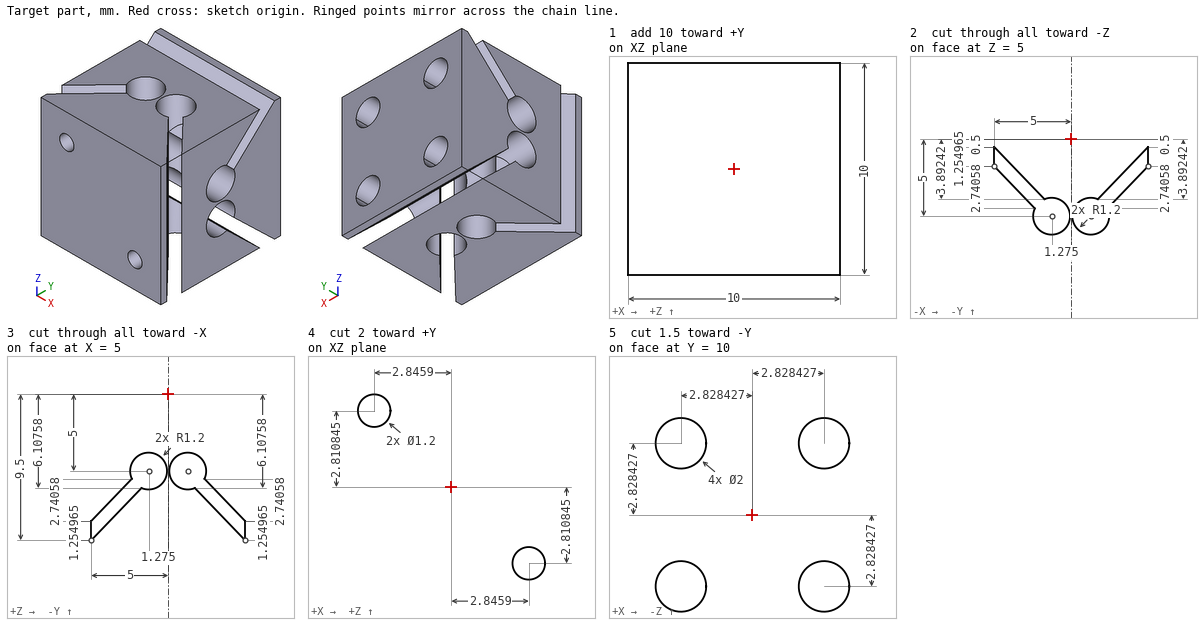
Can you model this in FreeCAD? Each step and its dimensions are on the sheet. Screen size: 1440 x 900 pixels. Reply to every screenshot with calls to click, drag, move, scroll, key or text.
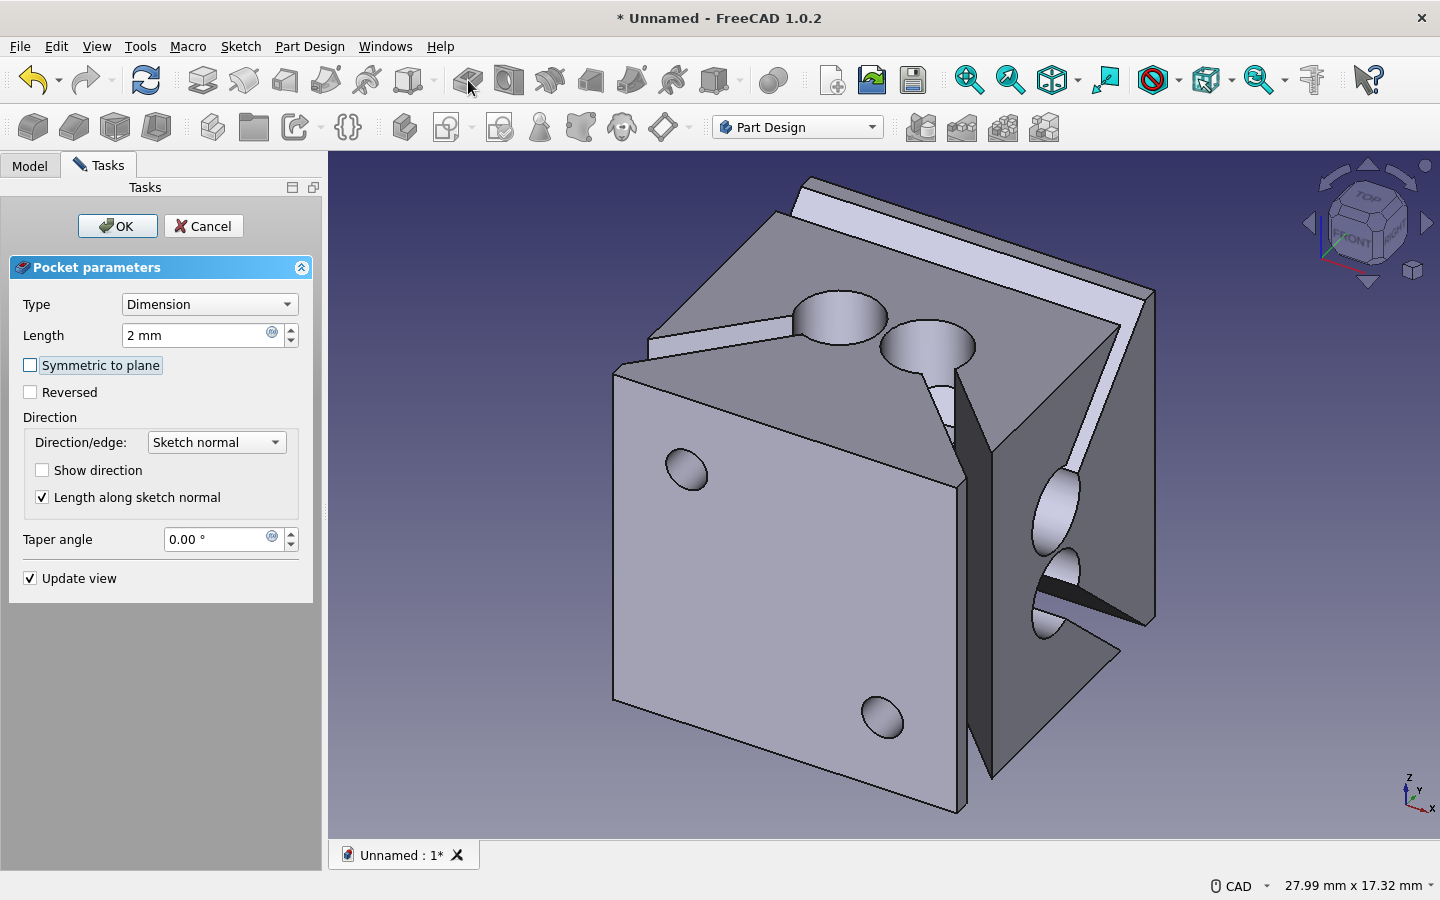
click(118, 226)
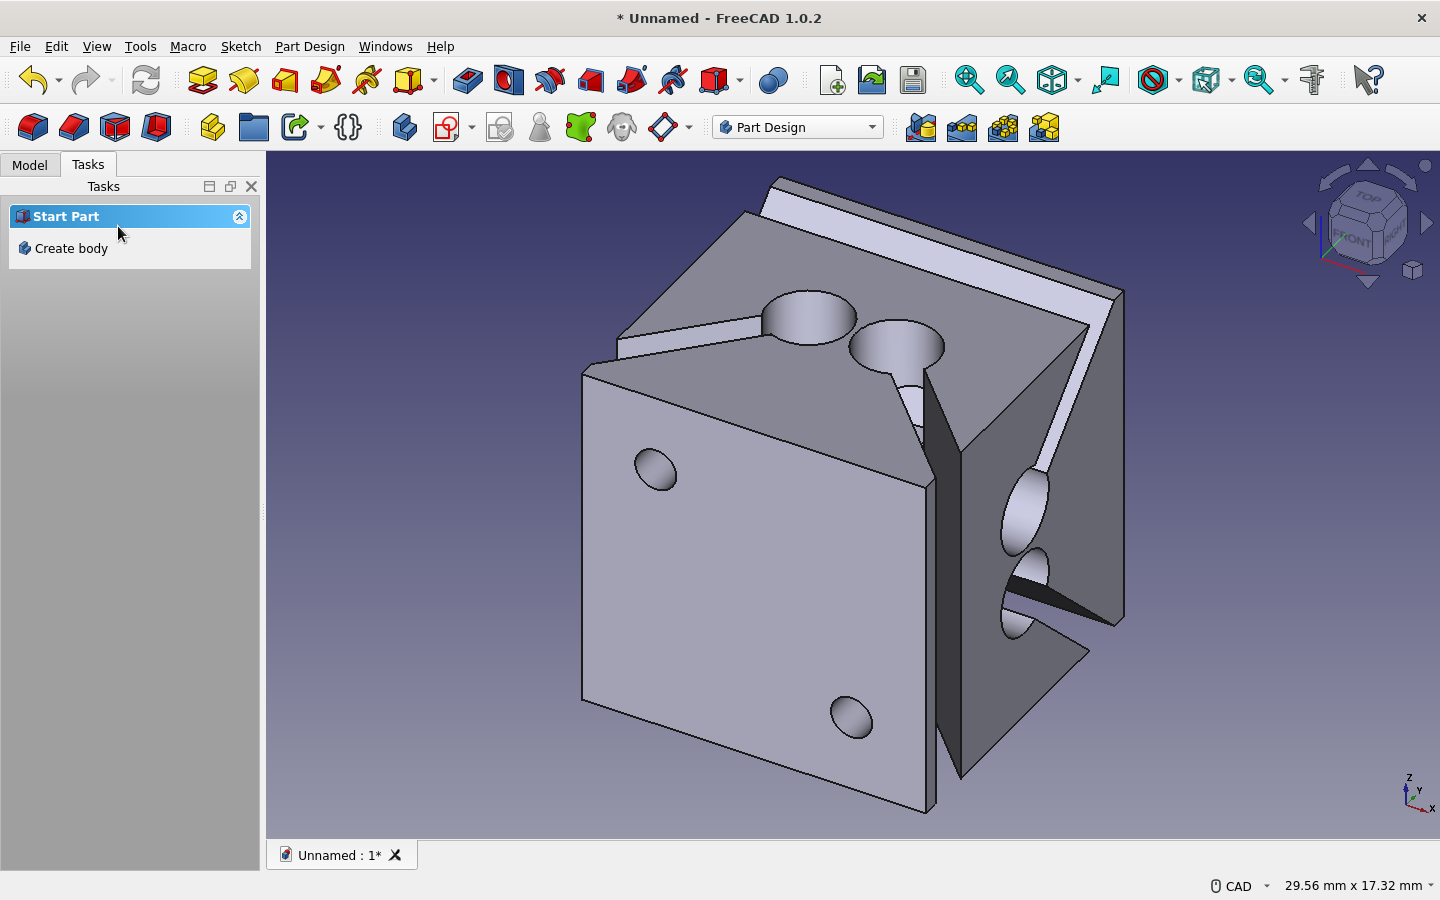
key(4)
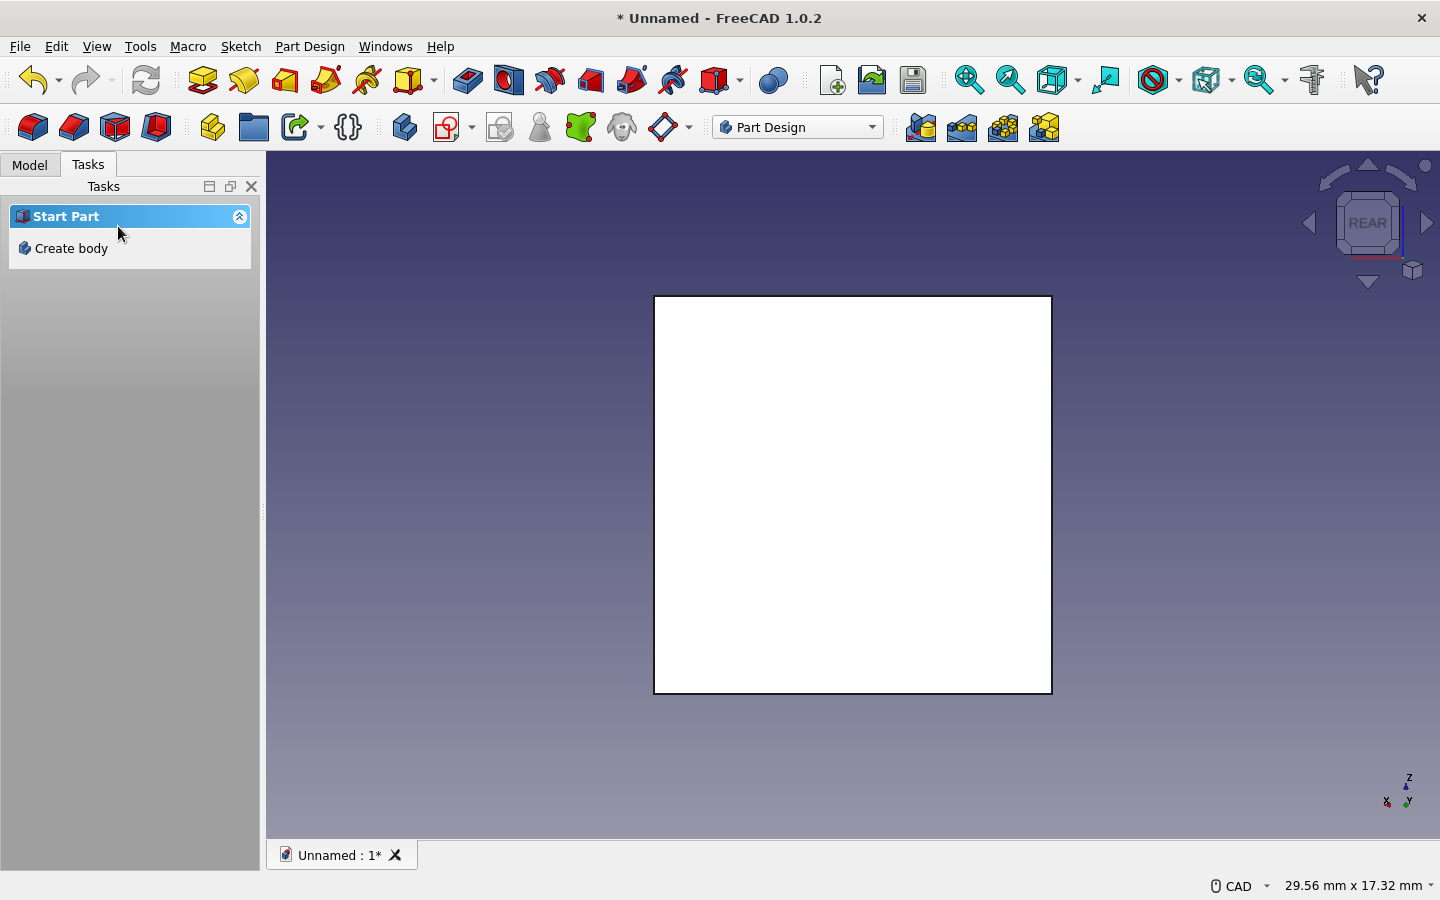
click(853, 494)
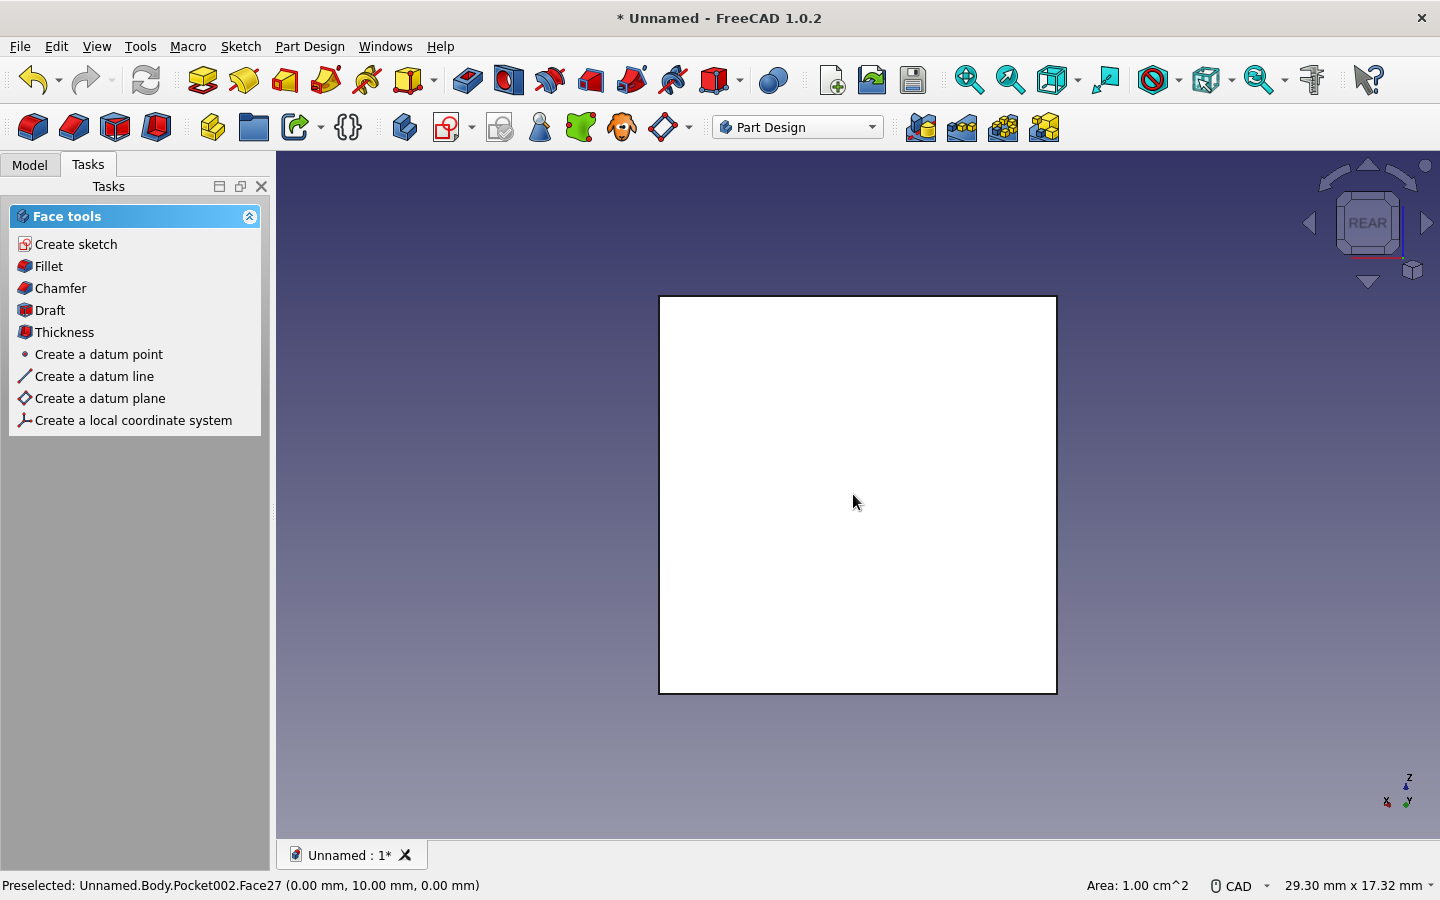
click(446, 128)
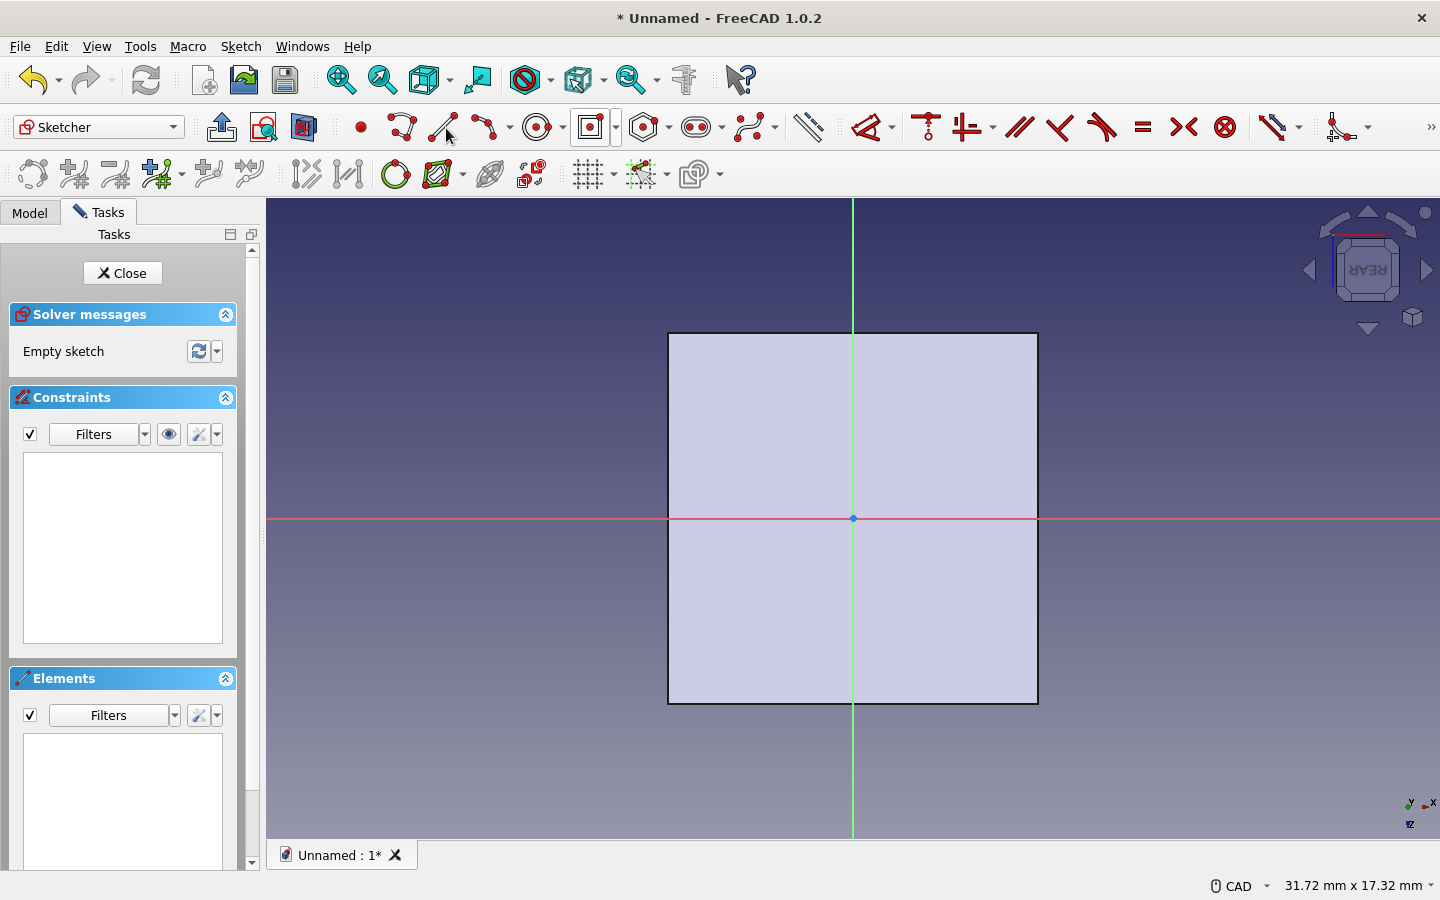
scroll(992, 518, up, 2)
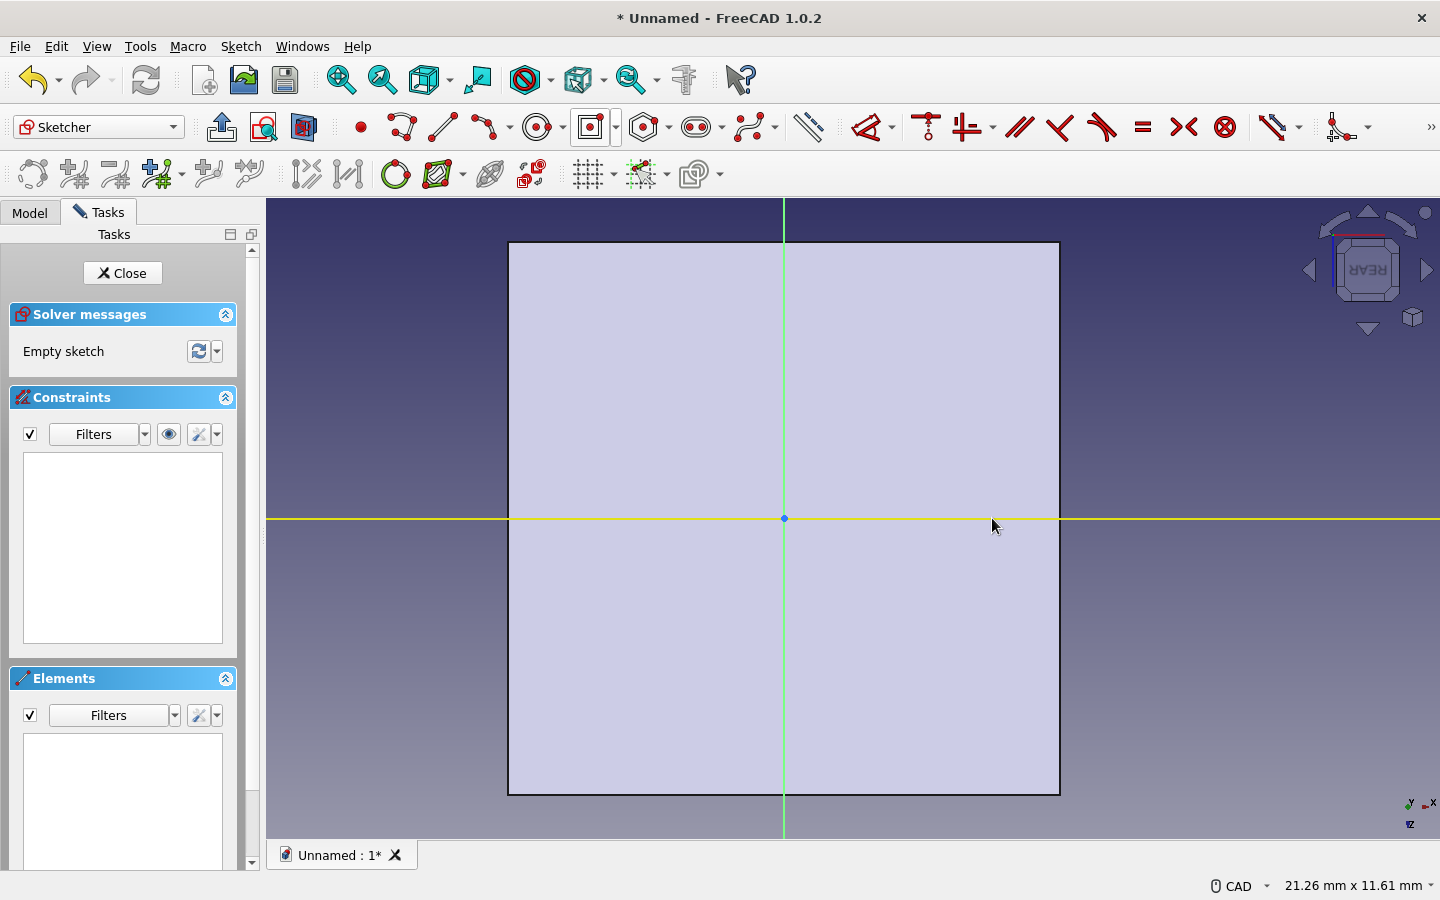
click(536, 128)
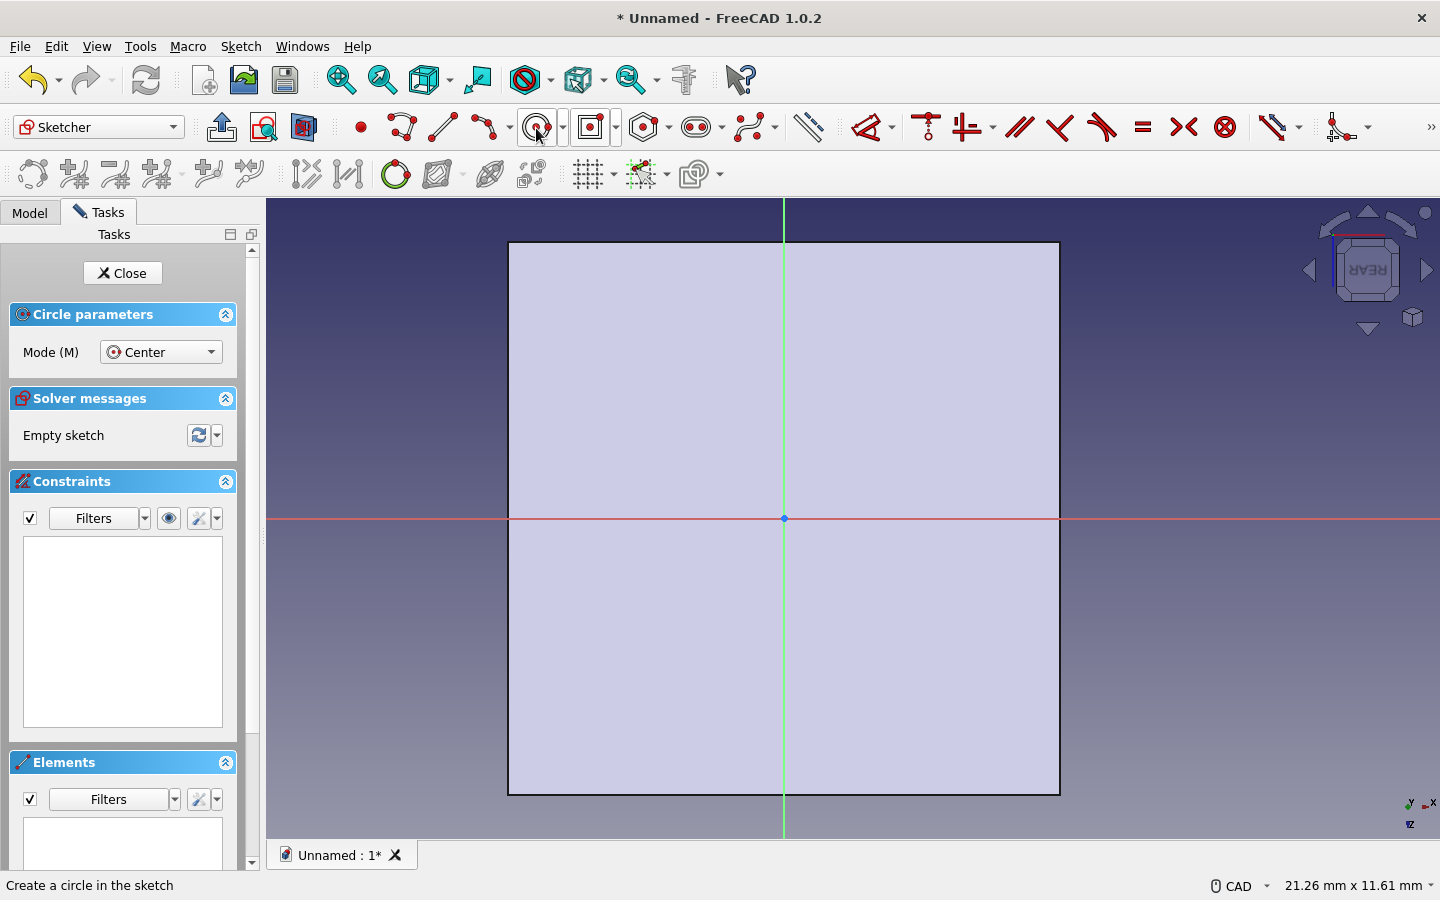
click(628, 362)
move(667, 323)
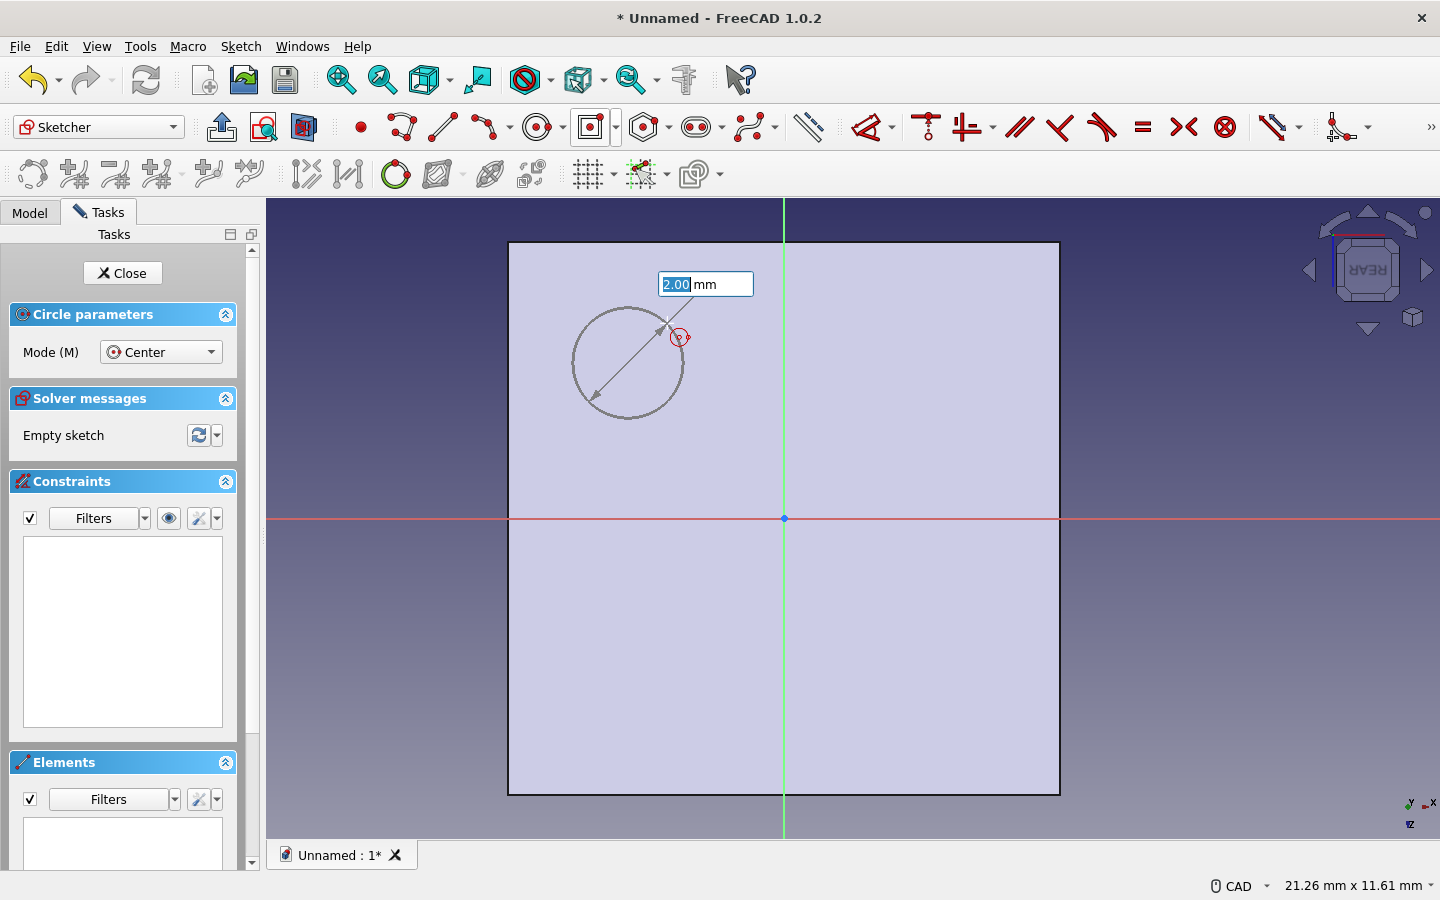
text(2)
key(Return)